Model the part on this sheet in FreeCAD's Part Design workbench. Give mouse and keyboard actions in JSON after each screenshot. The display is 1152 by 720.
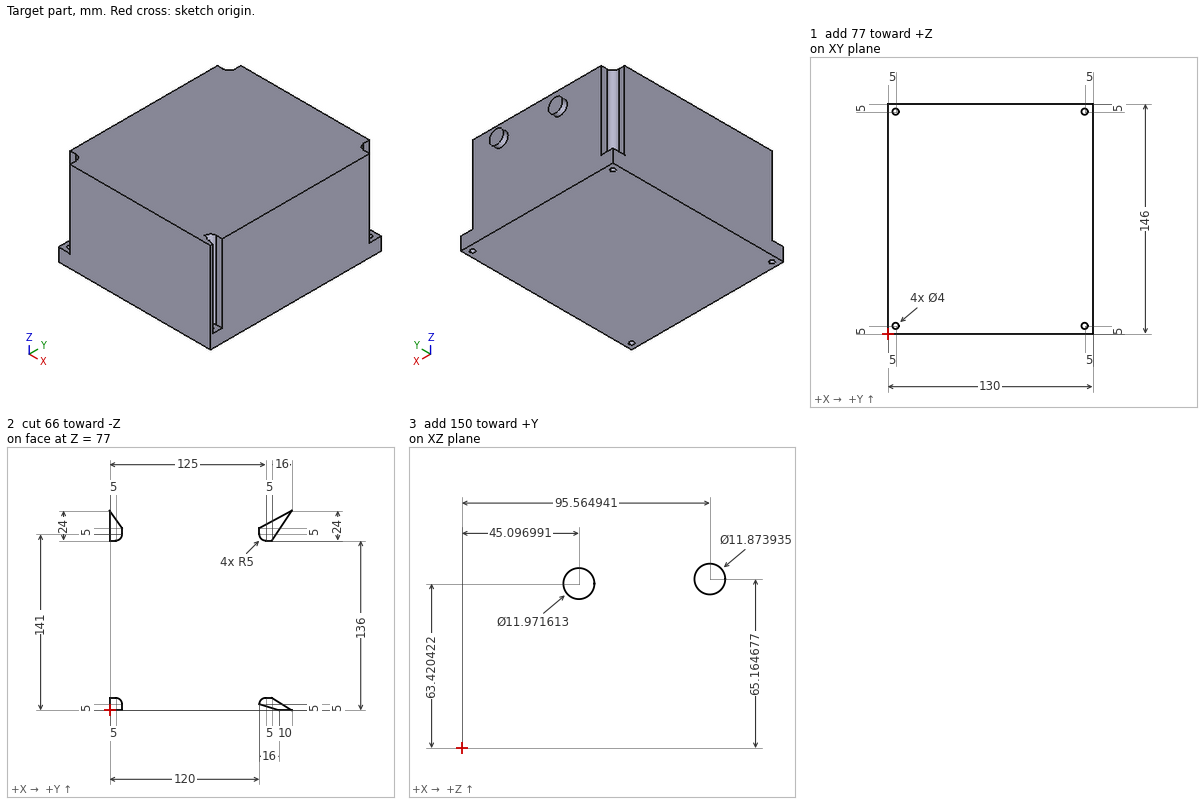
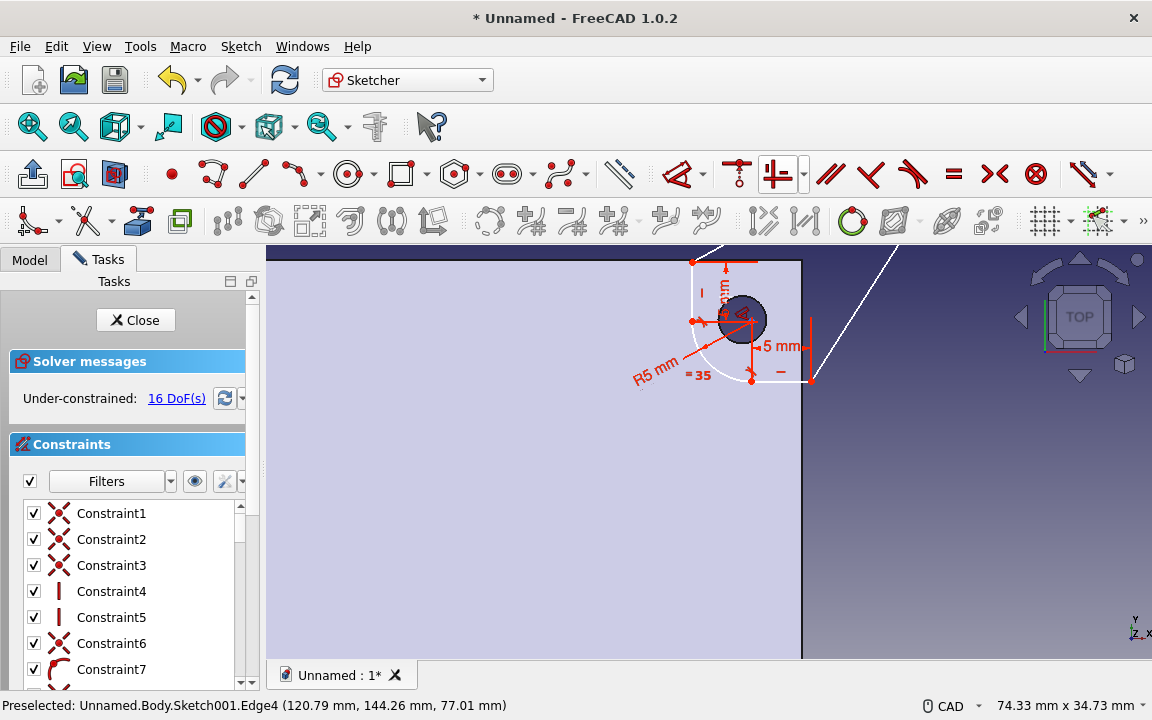
{"action": "scroll", "coordinate": [722, 359], "scroll_direction": "down", "scroll_amount": 10}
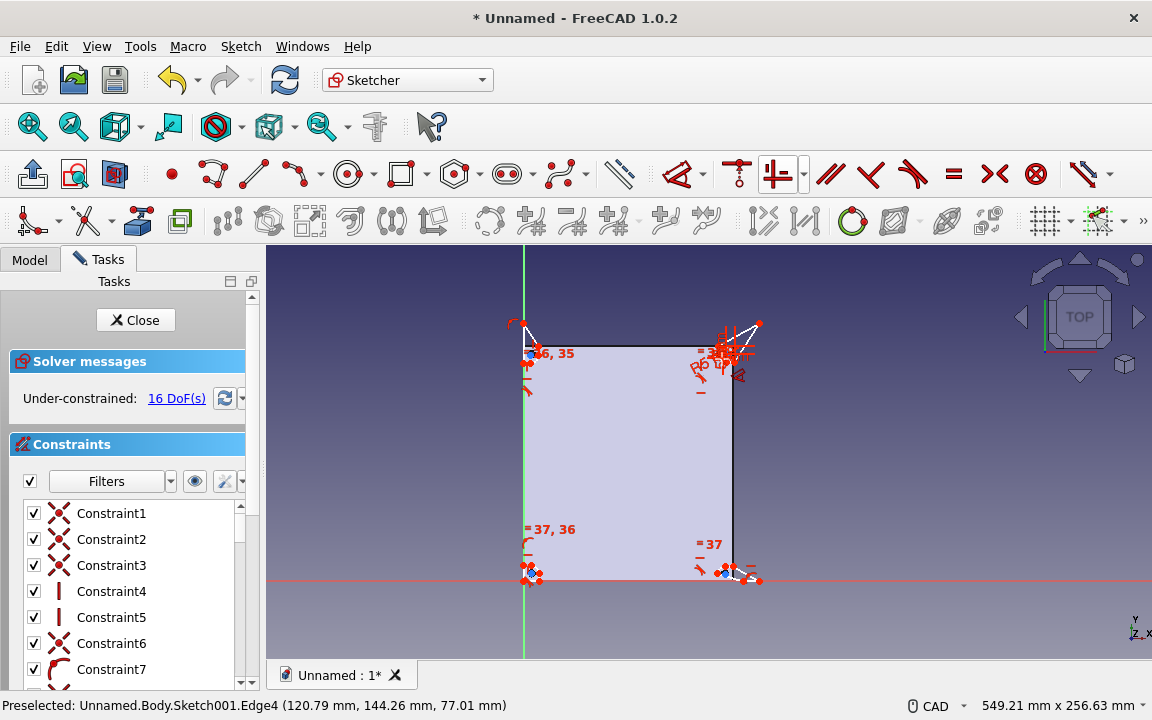
{"action": "scroll", "coordinate": [539, 353], "scroll_direction": "up", "scroll_amount": 9}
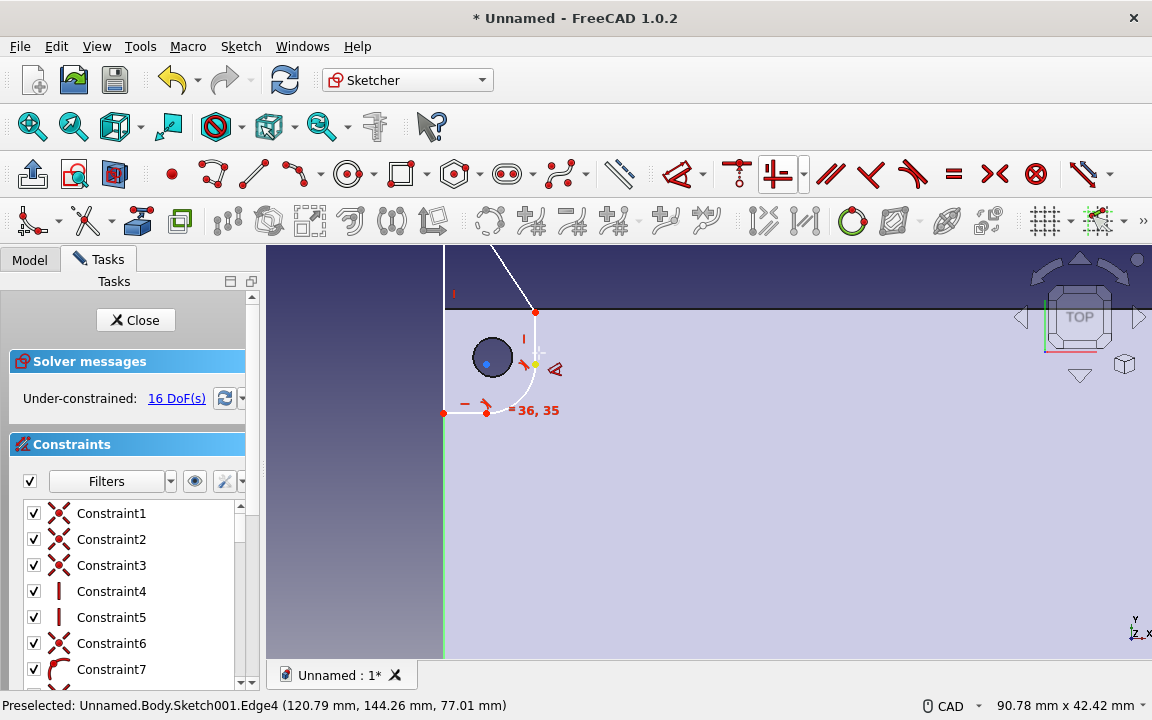
{"action": "left_click", "coordinate": [535, 349]}
{"action": "left_click", "coordinate": [501, 338]}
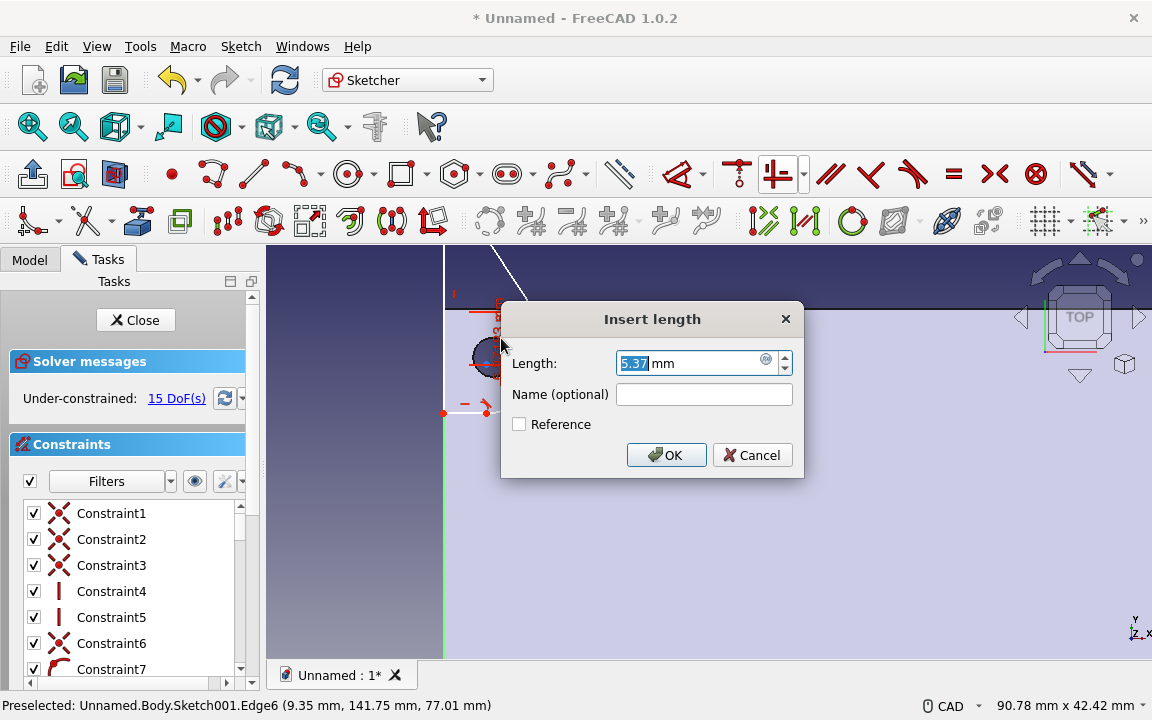
{"action": "type", "text": "5"}
{"action": "key", "text": "Return"}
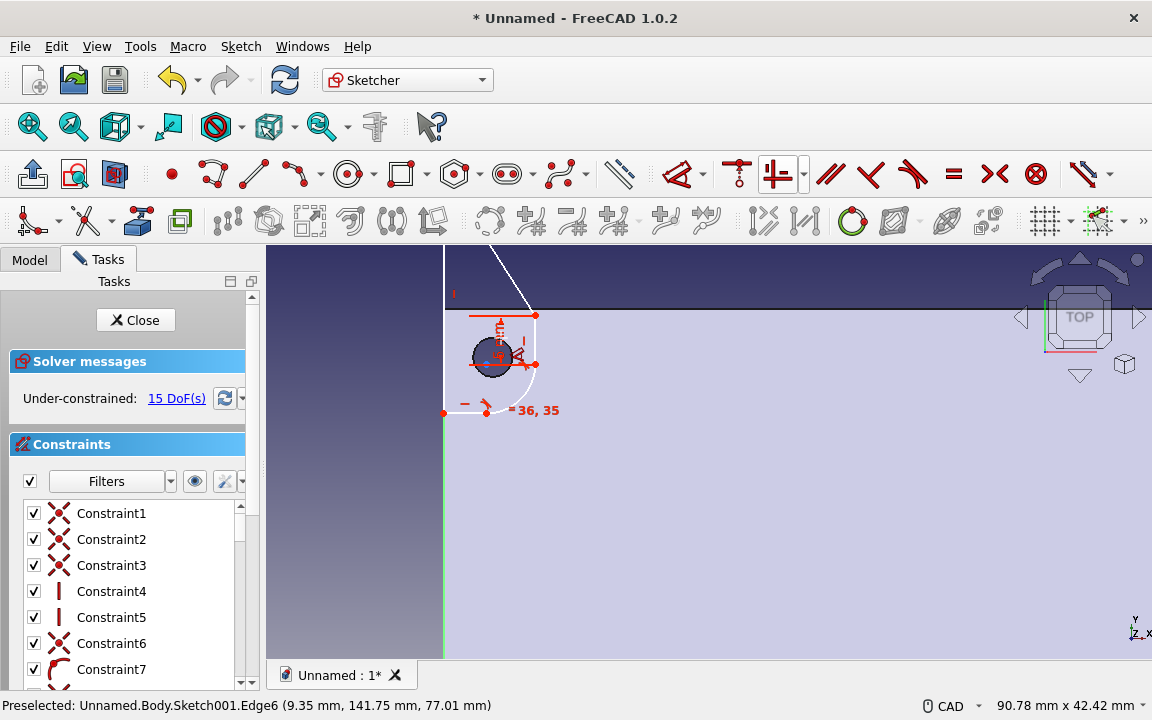
{"action": "left_click", "coordinate": [457, 413]}
{"action": "left_click", "coordinate": [465, 379]}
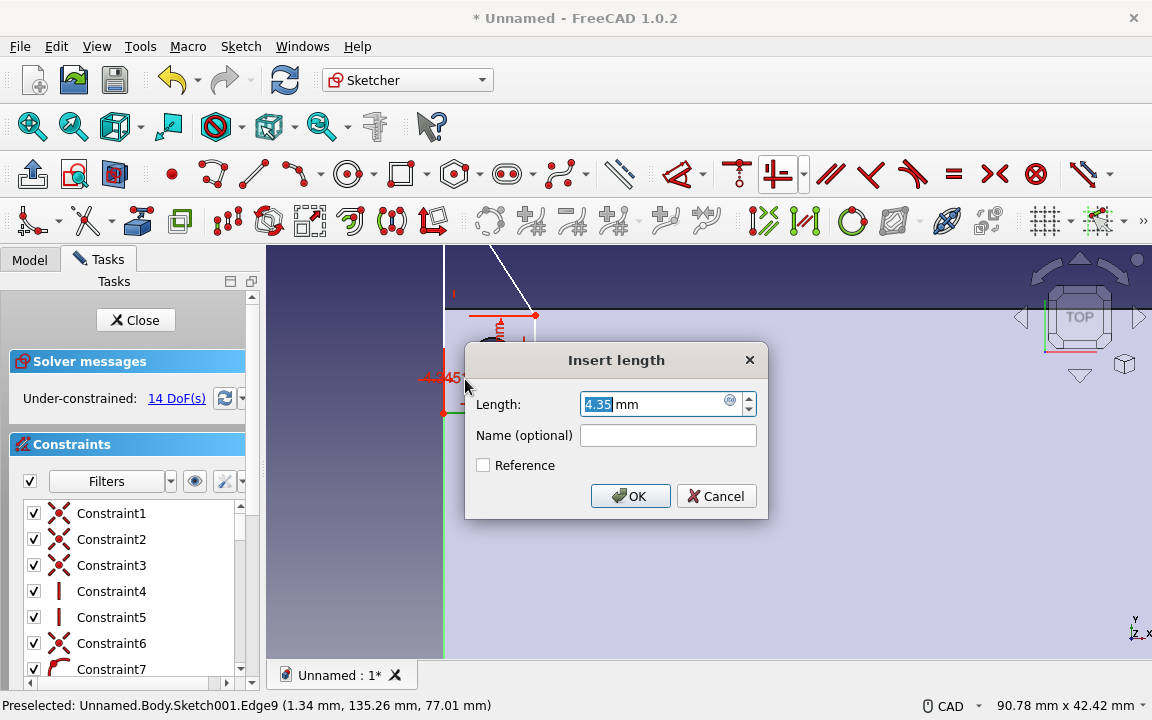
{"action": "type", "text": "5"}
{"action": "key", "text": "Return"}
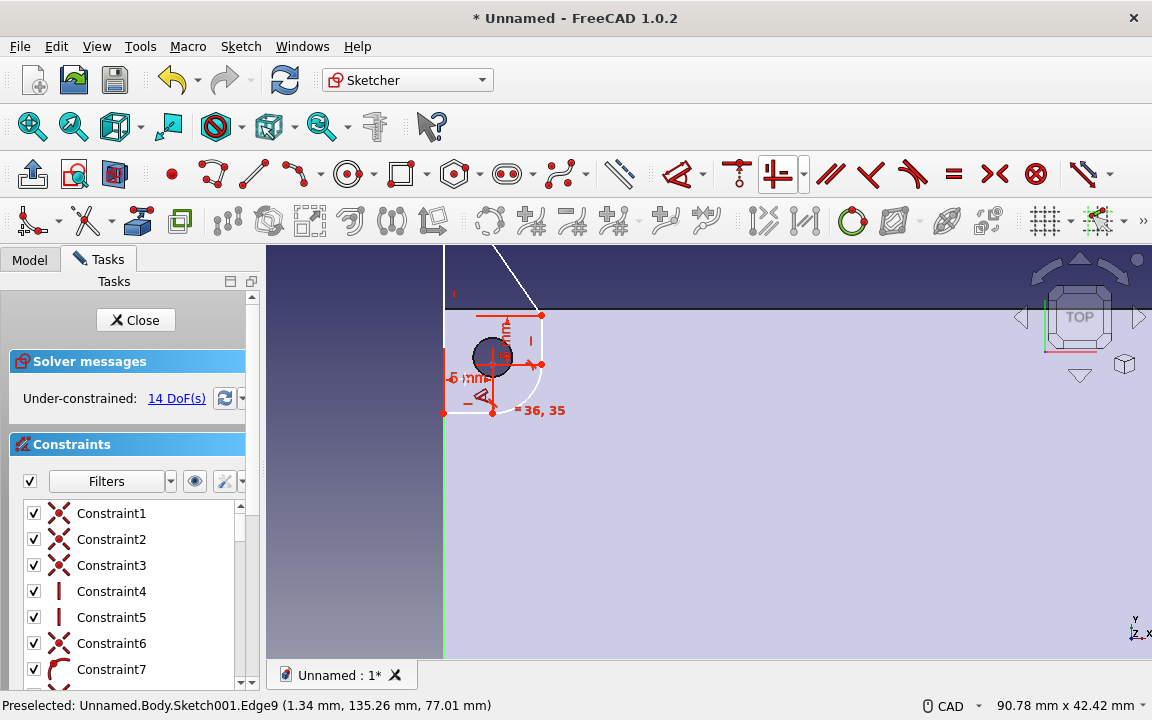
{"action": "scroll", "coordinate": [538, 353], "scroll_direction": "down", "scroll_amount": 9}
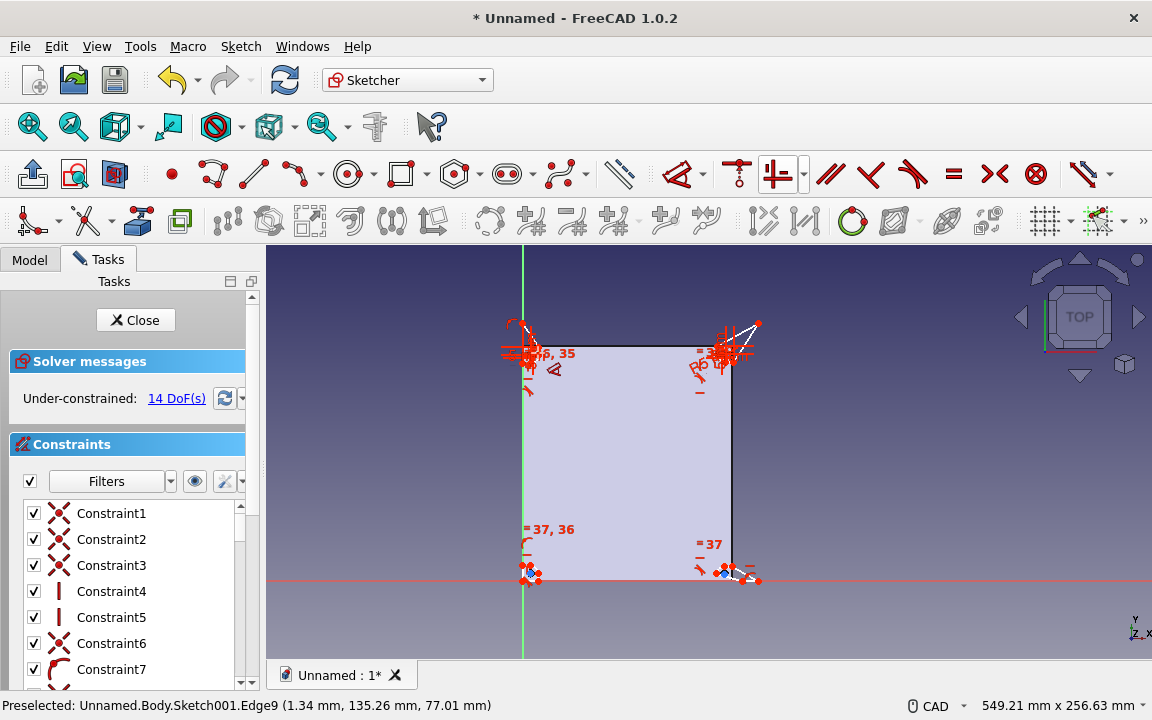
{"action": "scroll", "coordinate": [528, 566], "scroll_direction": "up", "scroll_amount": 10}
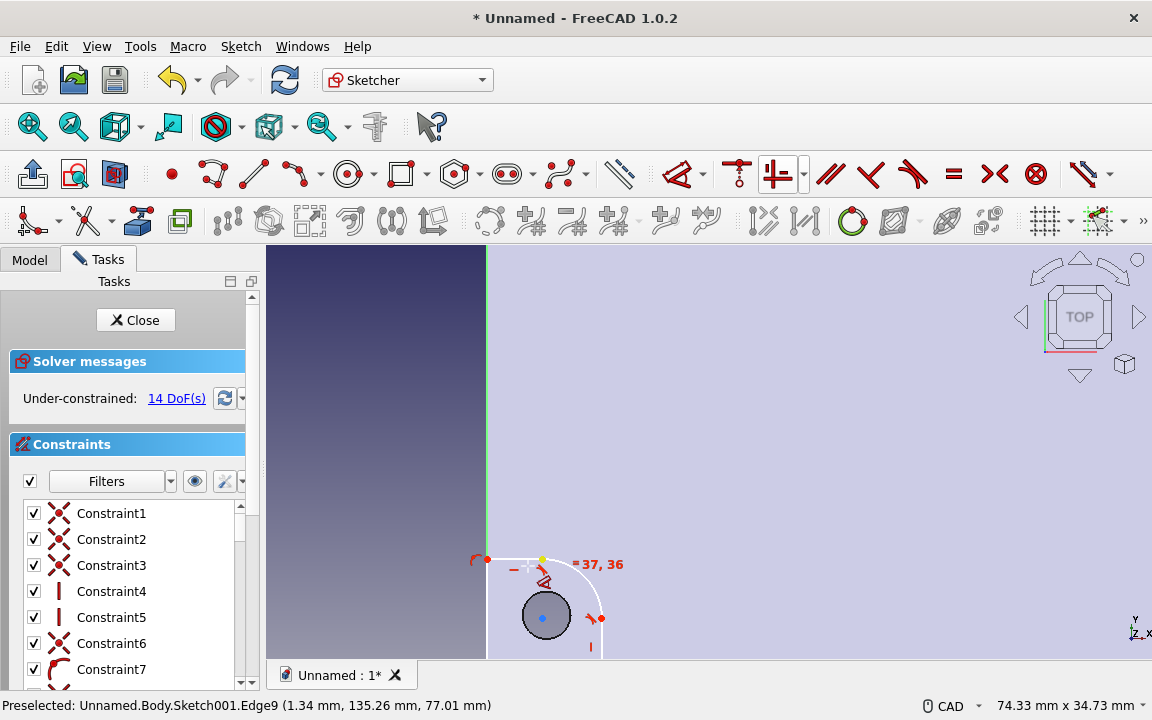
{"action": "left_click", "coordinate": [526, 559]}
{"action": "left_click", "coordinate": [515, 593]}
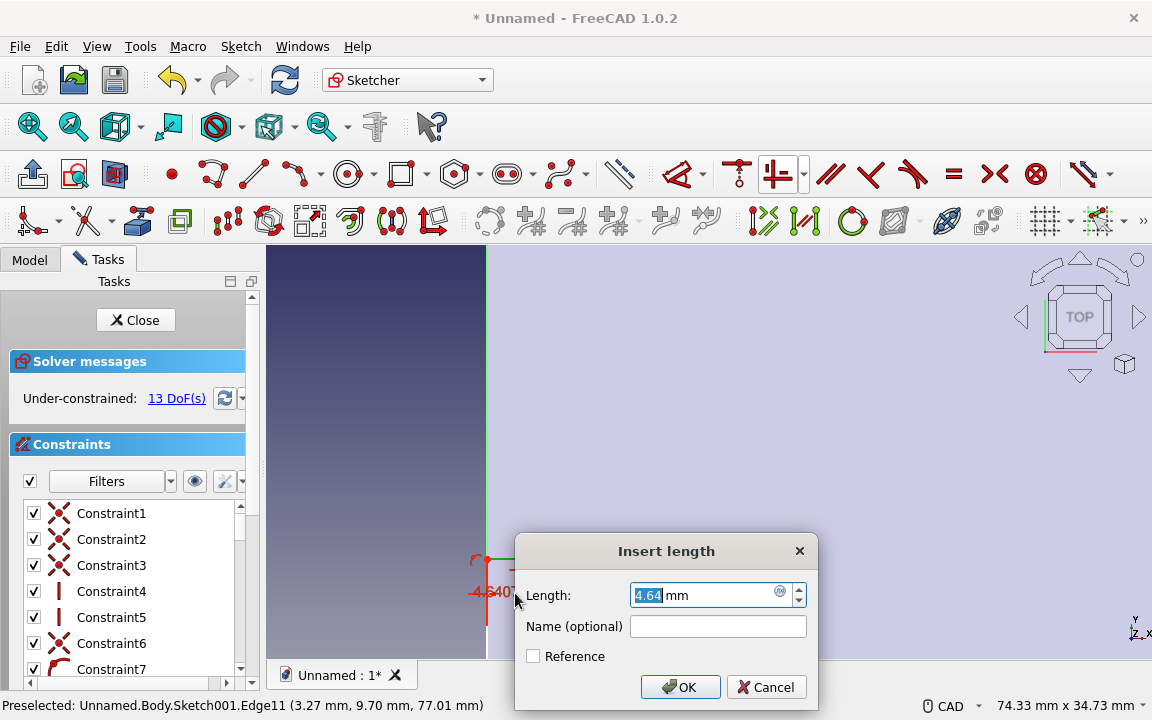
{"action": "type", "text": "5"}
{"action": "key", "text": "Return"}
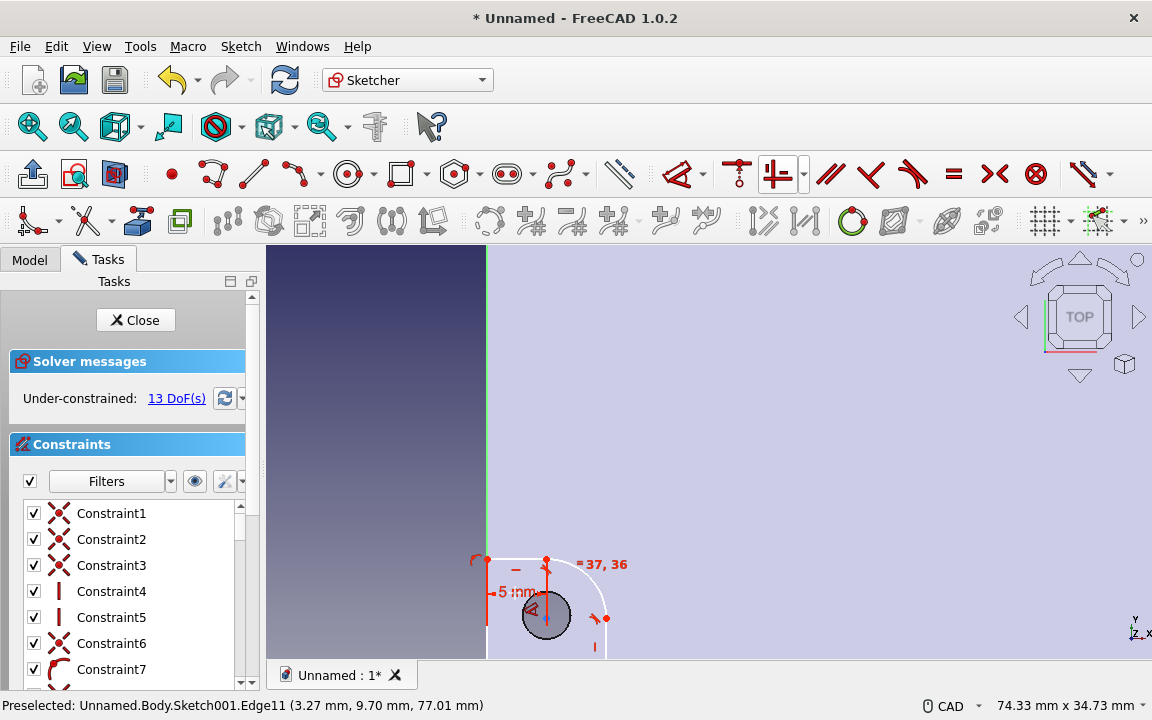
{"action": "scroll", "coordinate": [606, 630], "scroll_direction": "up", "scroll_amount": 2}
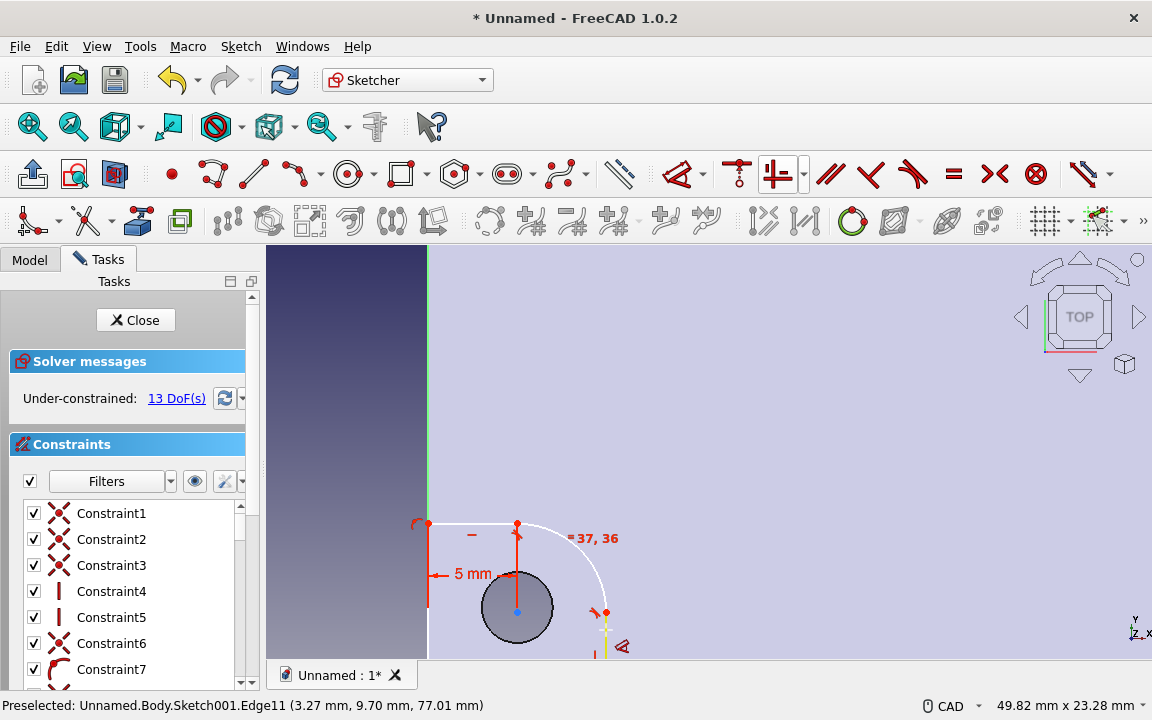
{"action": "left_click", "coordinate": [606, 630]}
{"action": "left_click", "coordinate": [572, 622]}